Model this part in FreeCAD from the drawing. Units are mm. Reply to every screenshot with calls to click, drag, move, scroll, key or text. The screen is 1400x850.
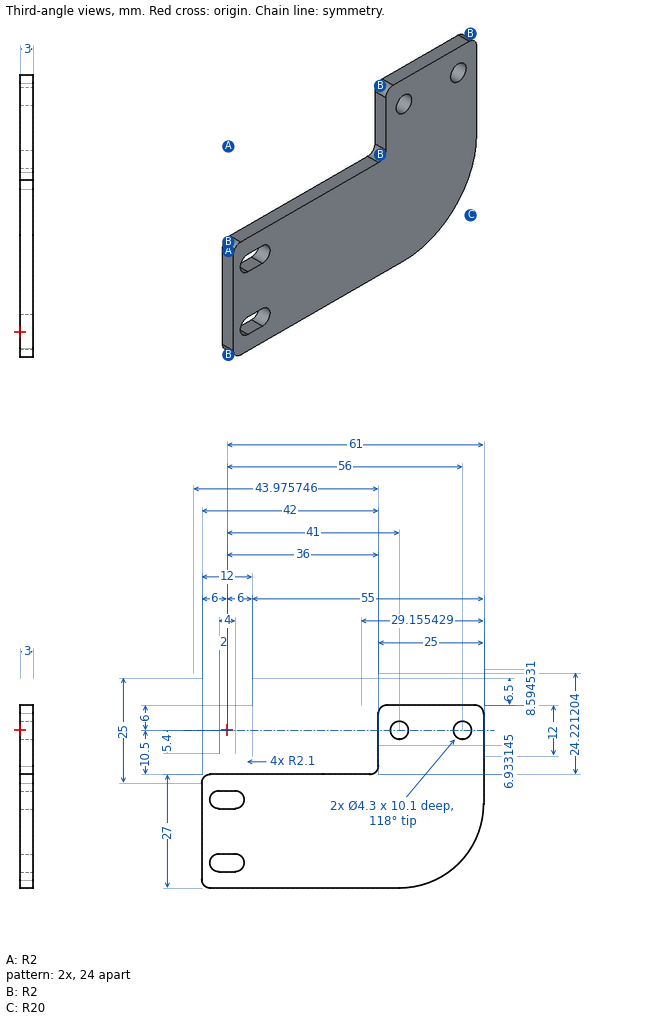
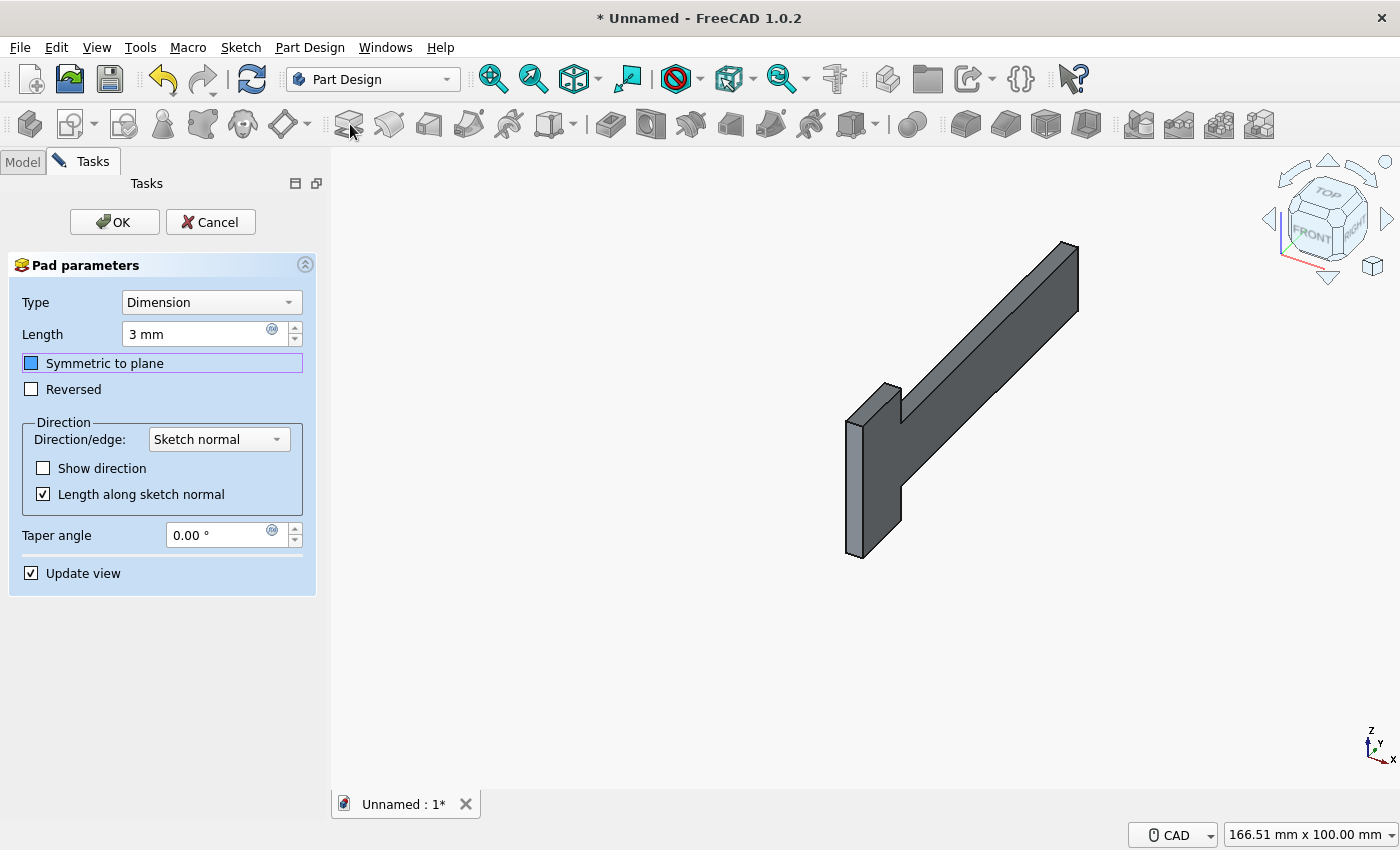
click(115, 222)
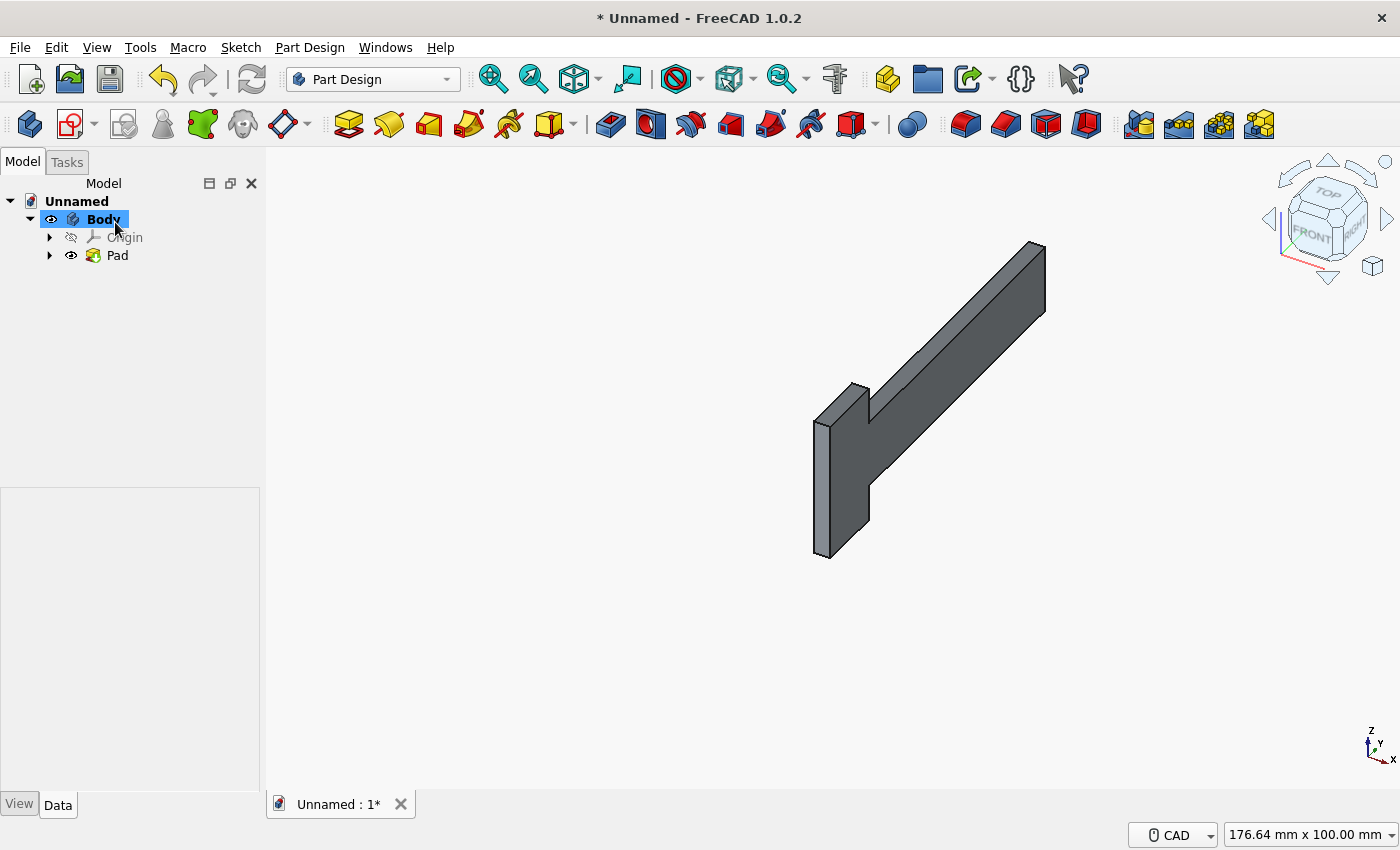
click(70, 124)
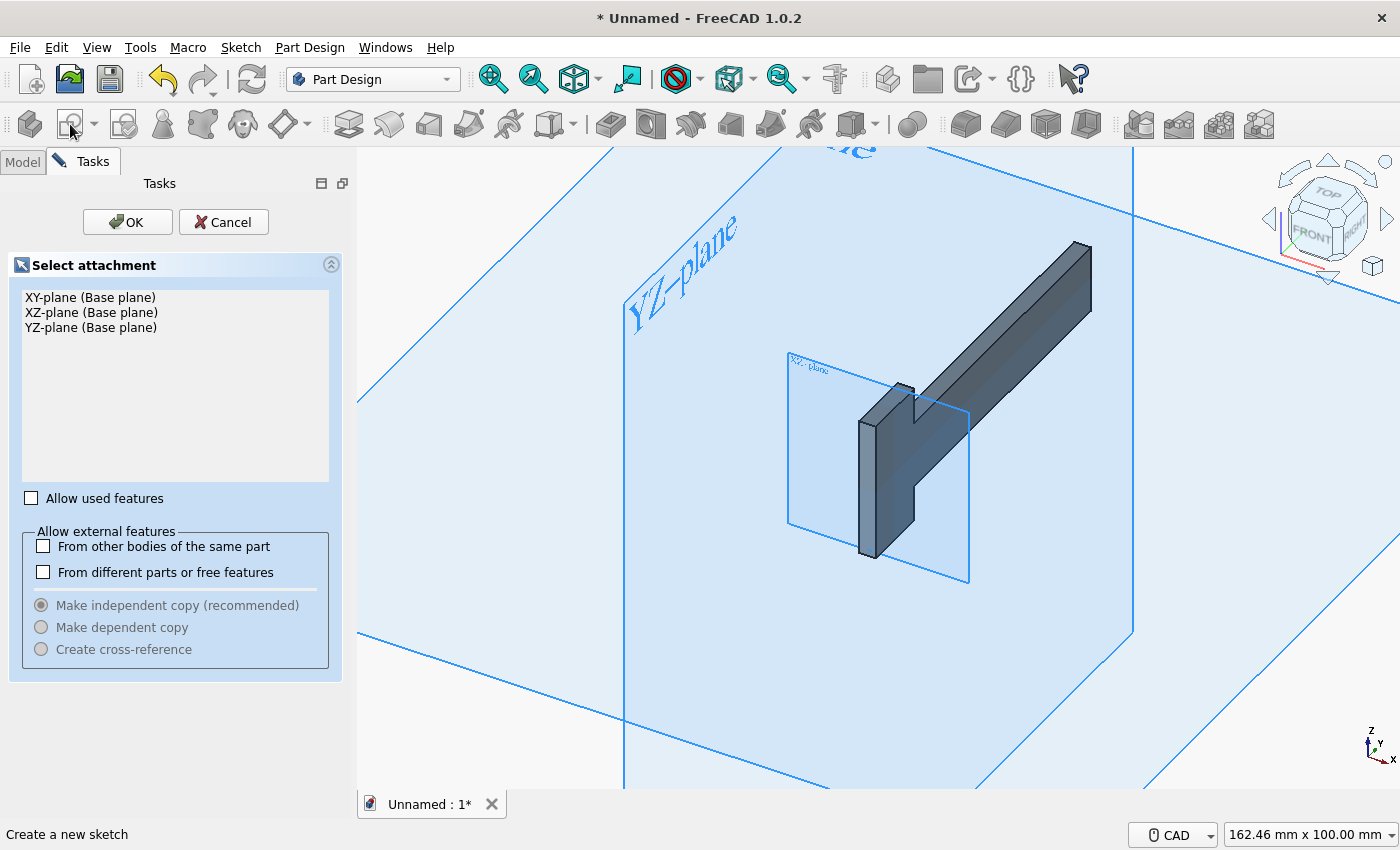
click(82, 328)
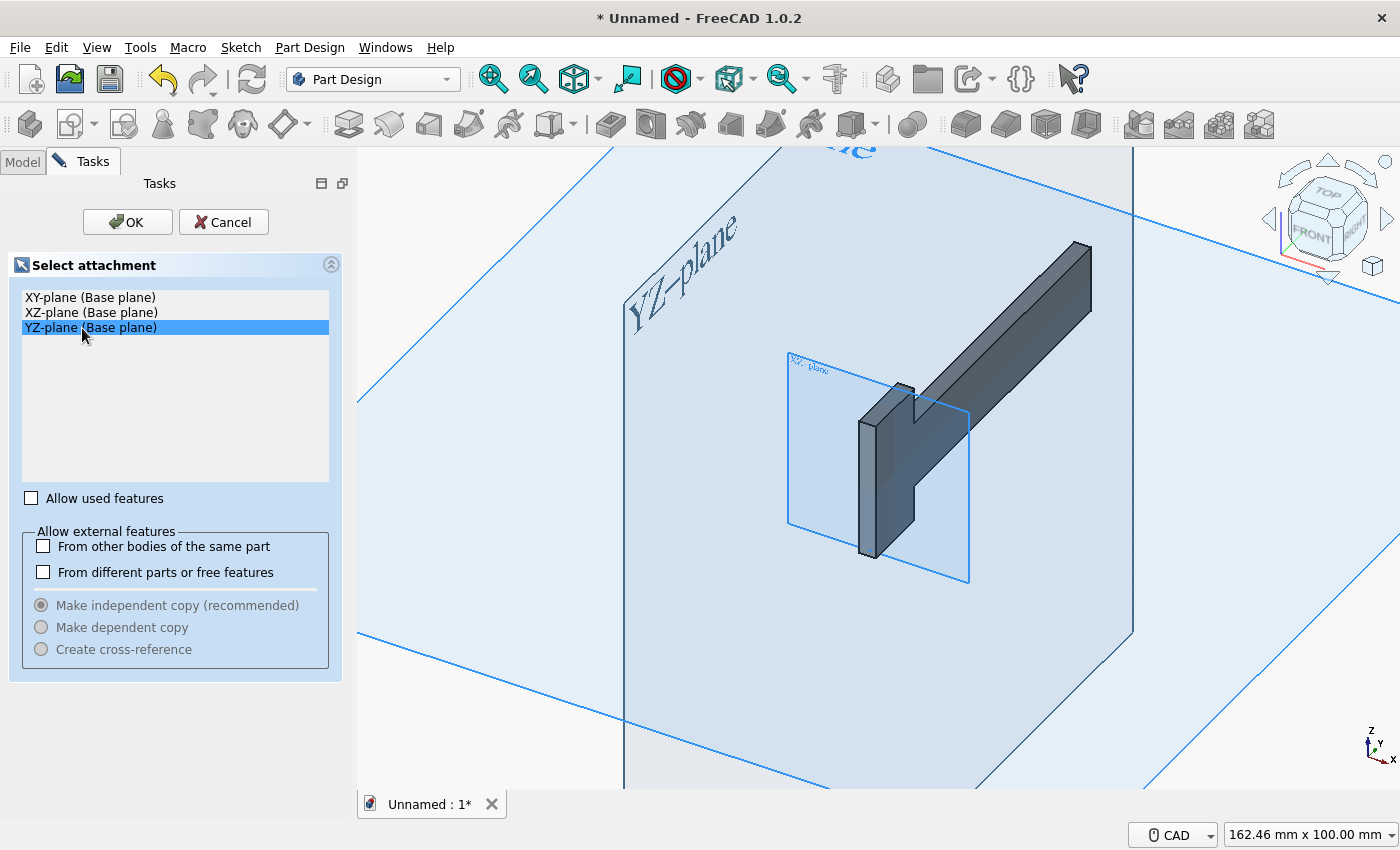
click(128, 222)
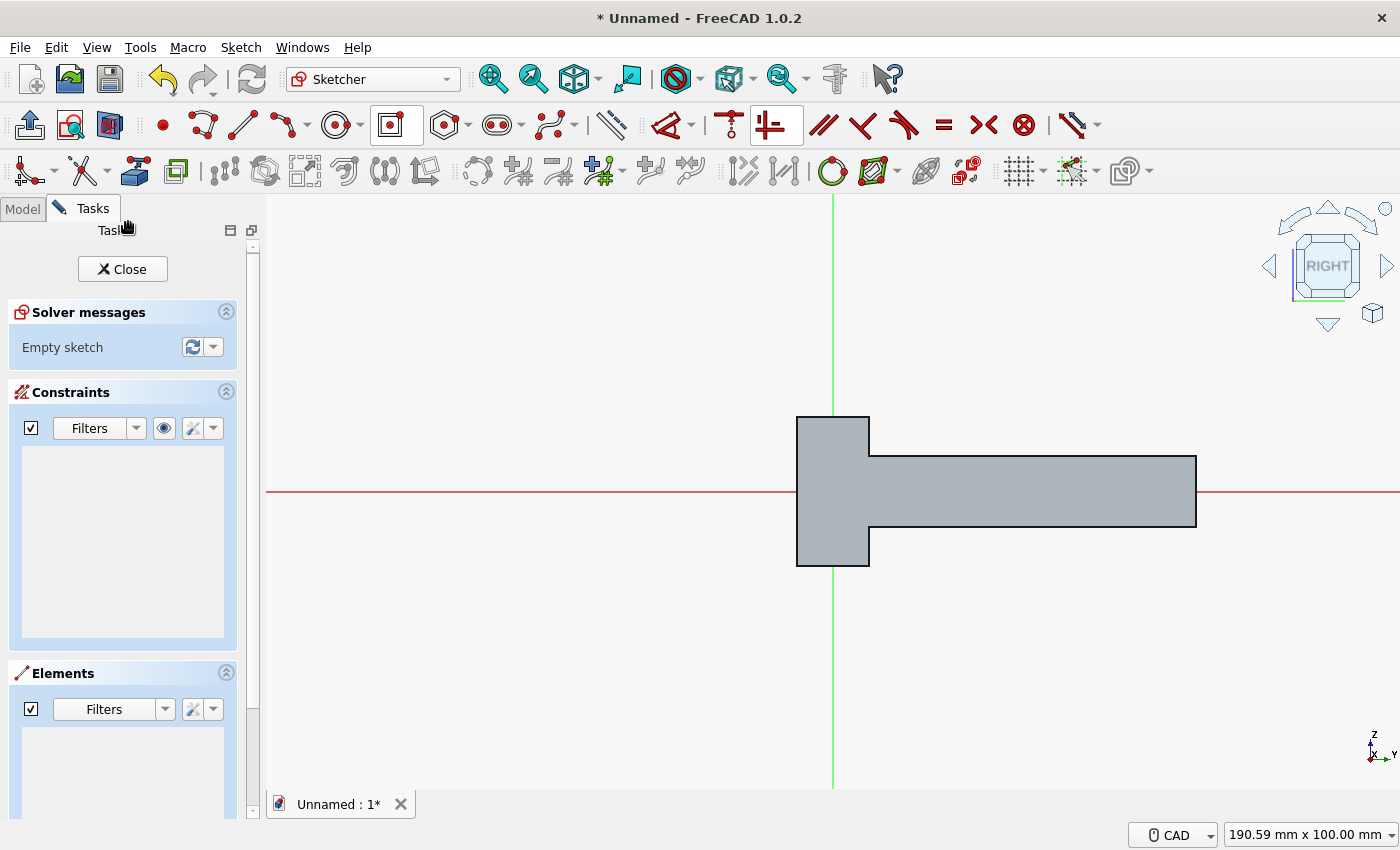
click(110, 126)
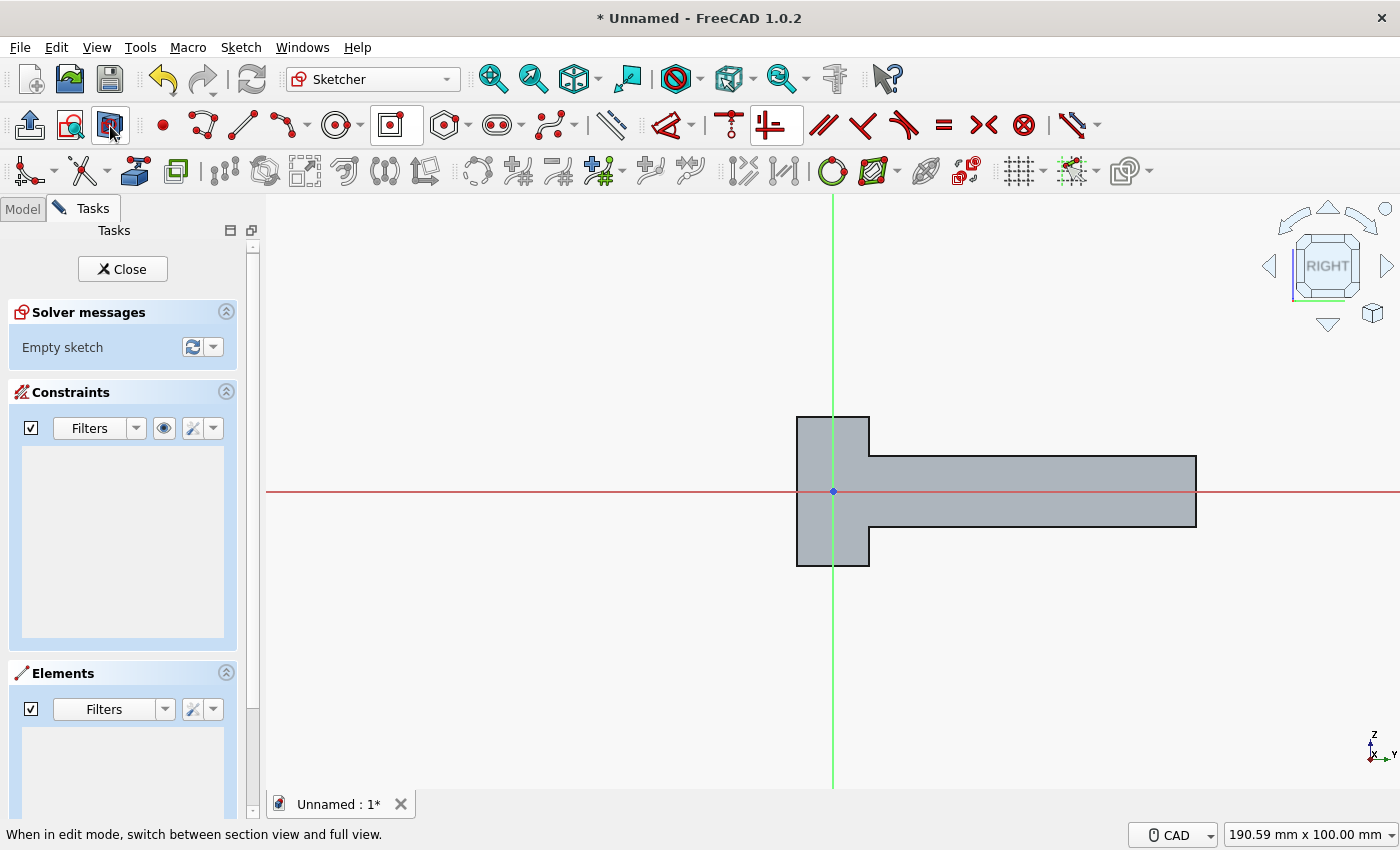
scroll(1235, 492, up, 3)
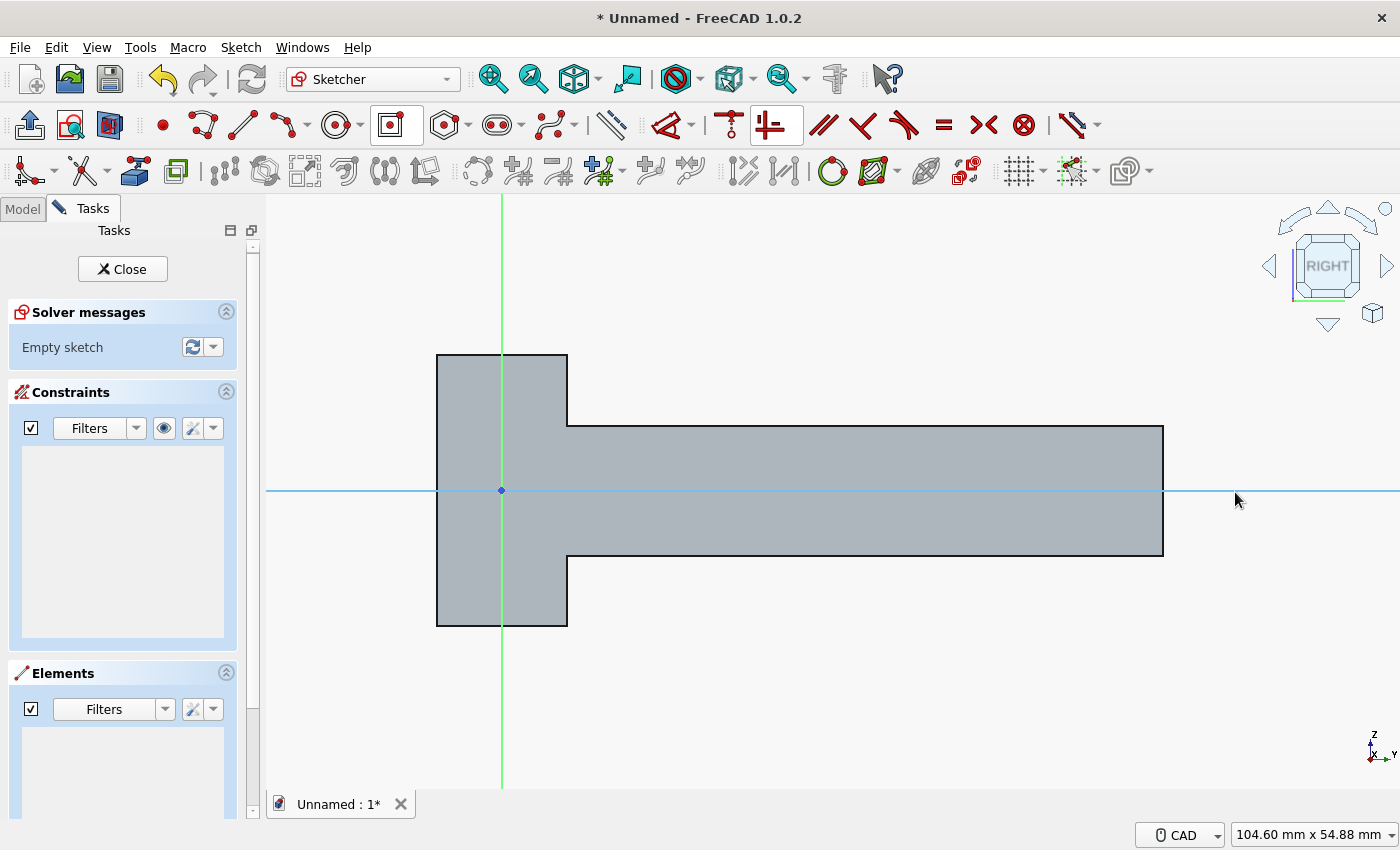
key(g)
key(m)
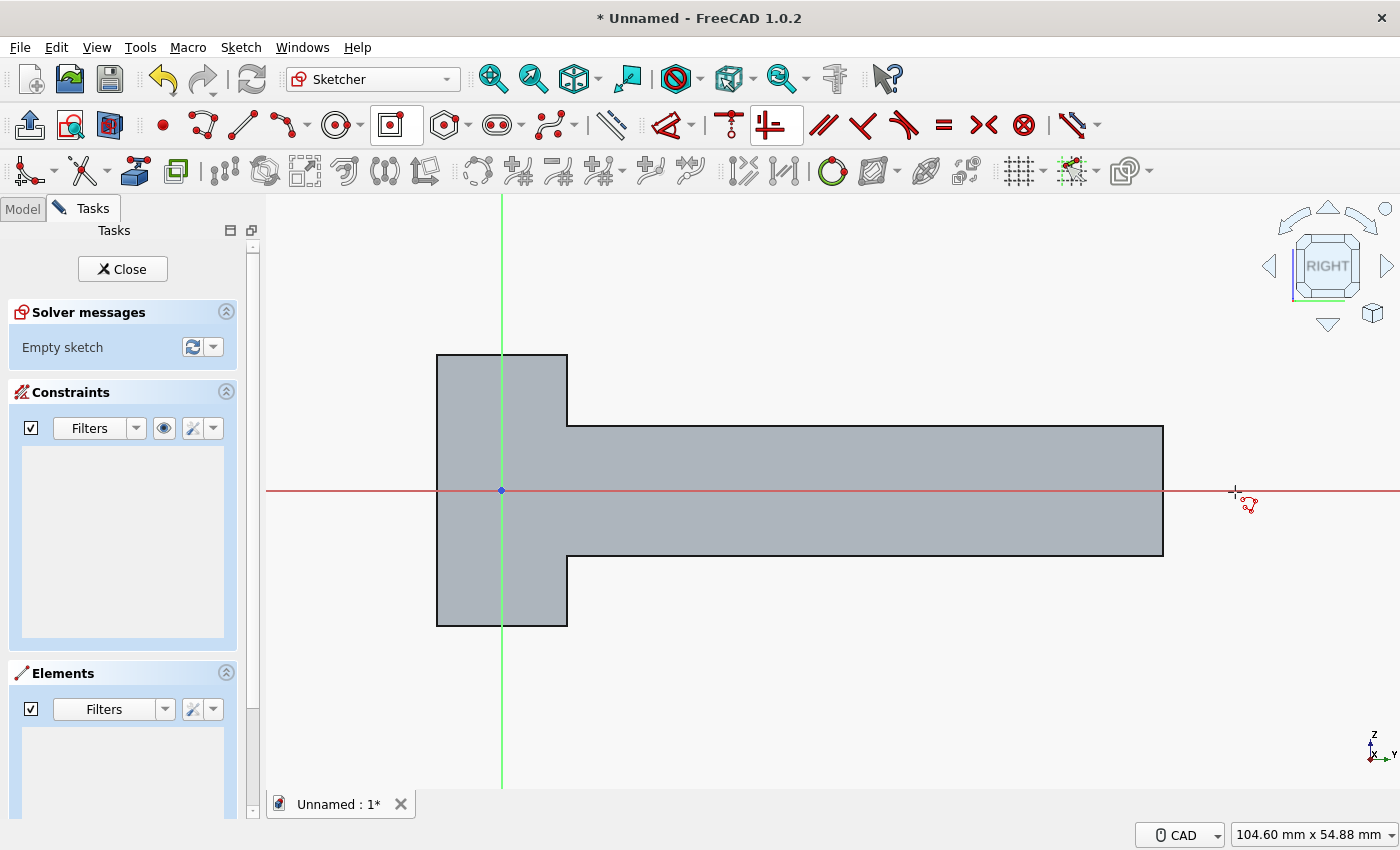
click(567, 626)
click(567, 355)
click(1163, 426)
click(1163, 556)
click(567, 627)
key(Escape)
key(Escape)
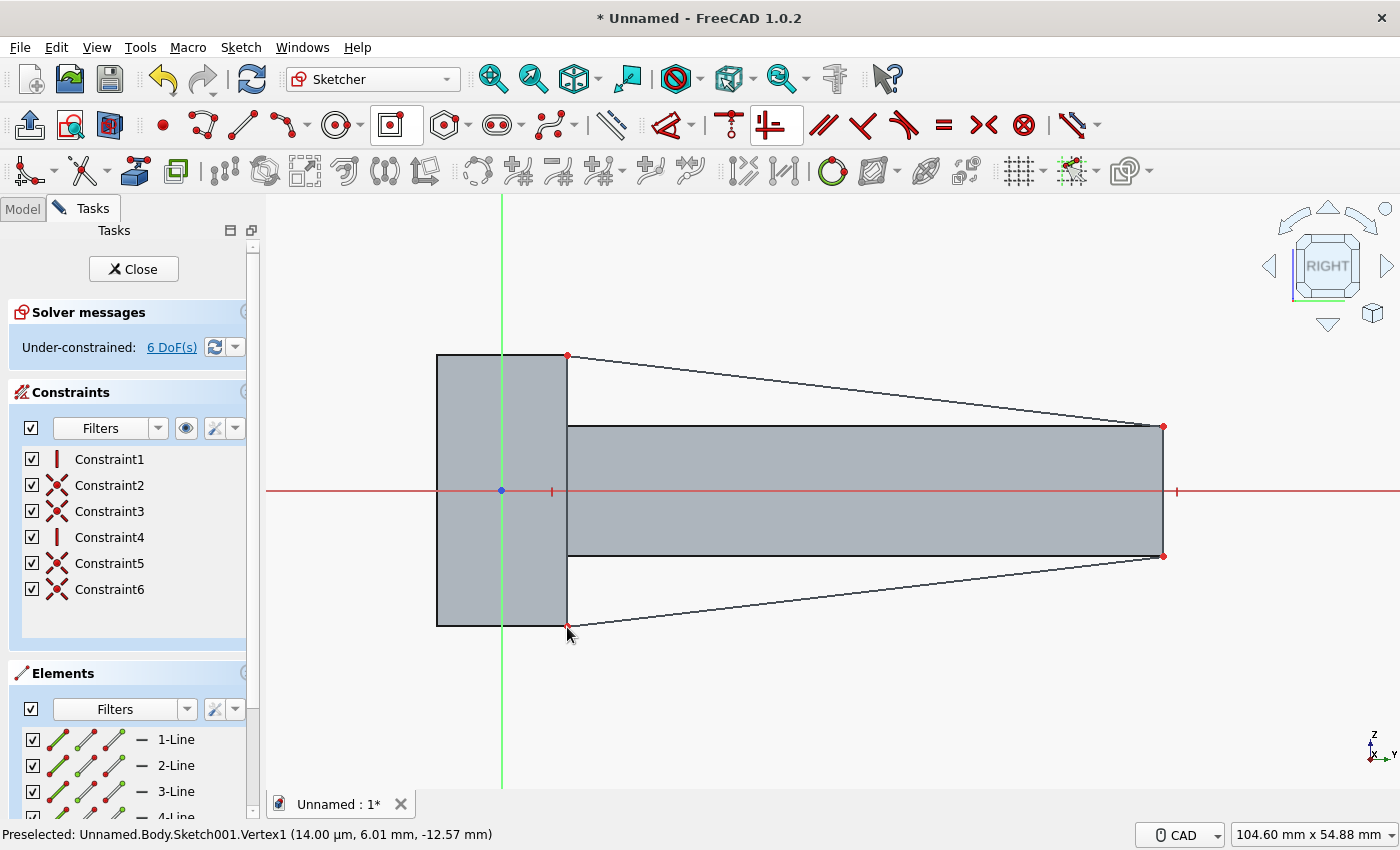
click(666, 126)